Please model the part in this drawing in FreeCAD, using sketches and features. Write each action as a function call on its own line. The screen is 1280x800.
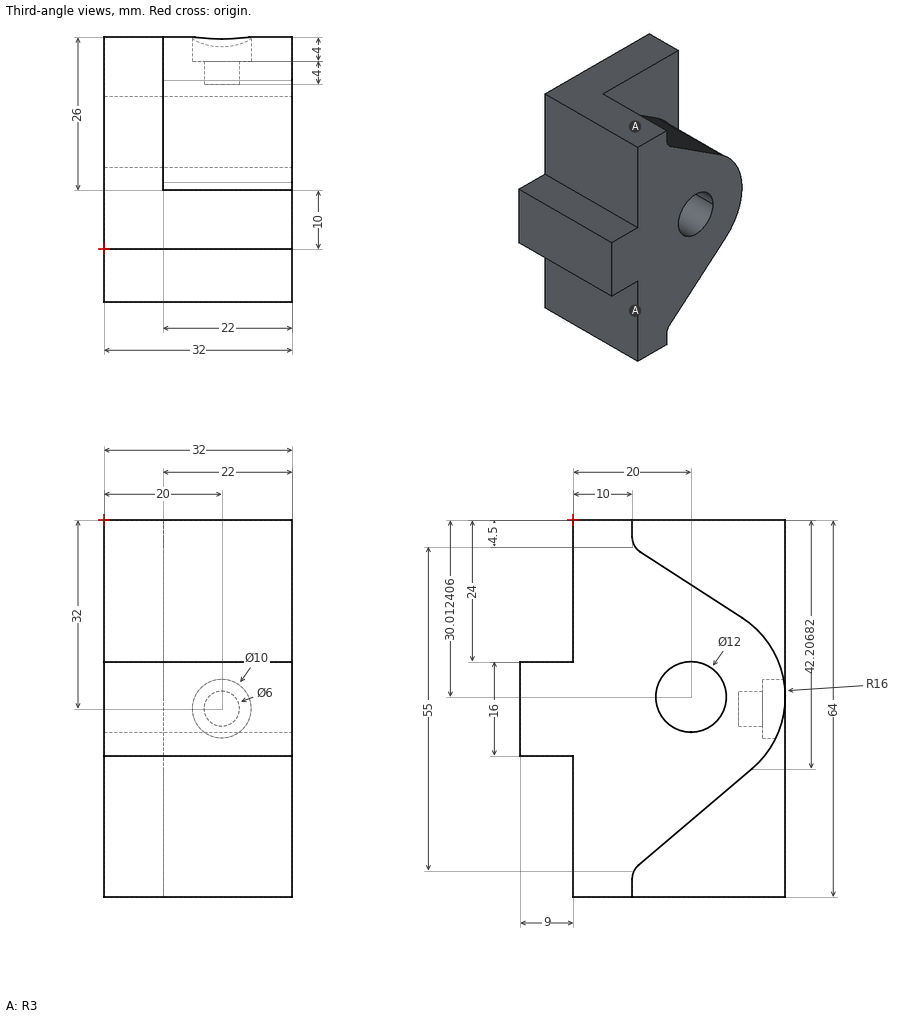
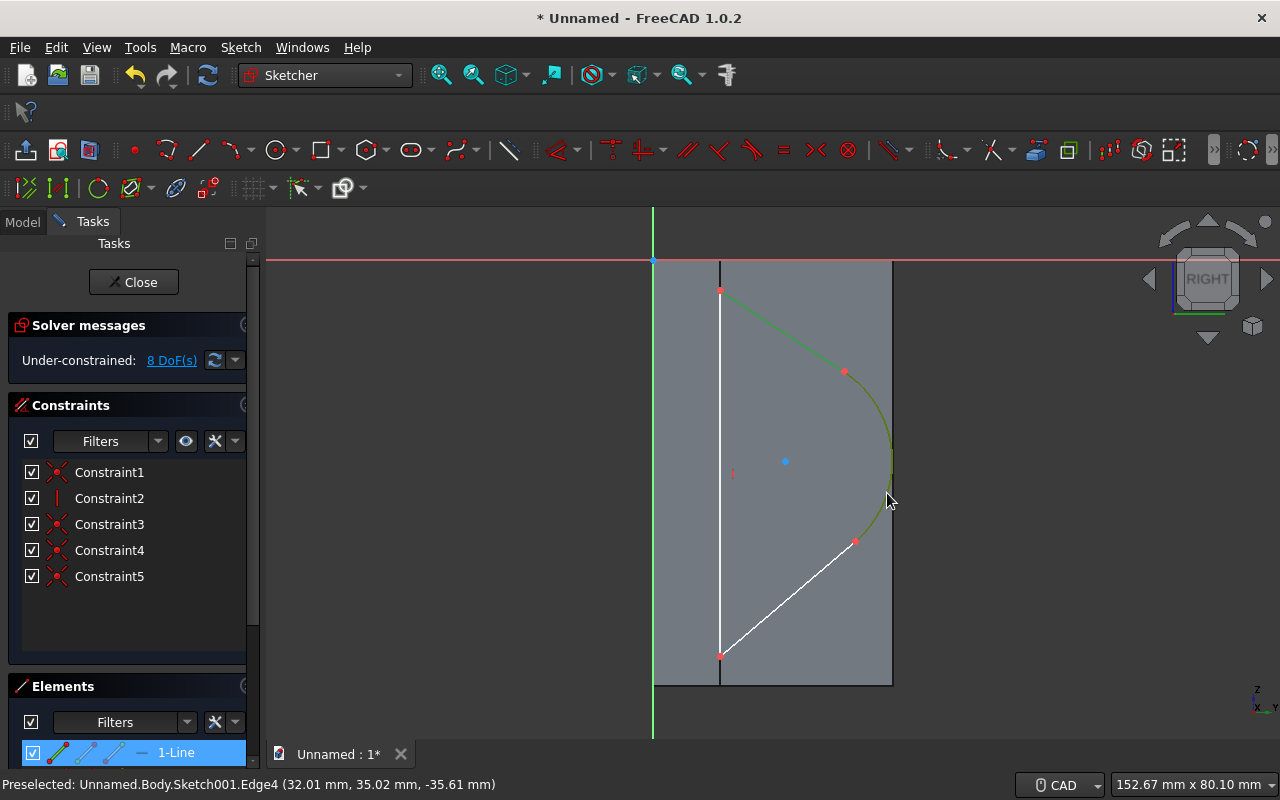
key(t)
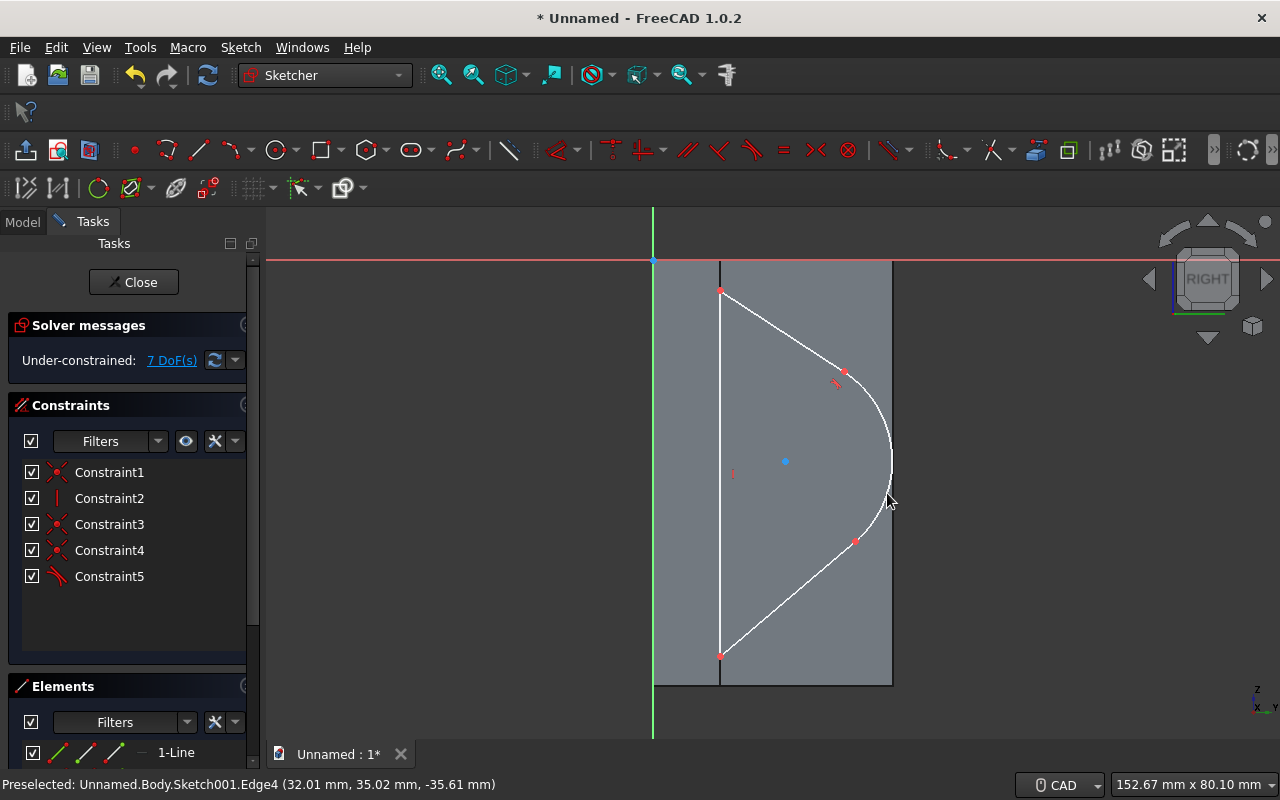
click(760, 623)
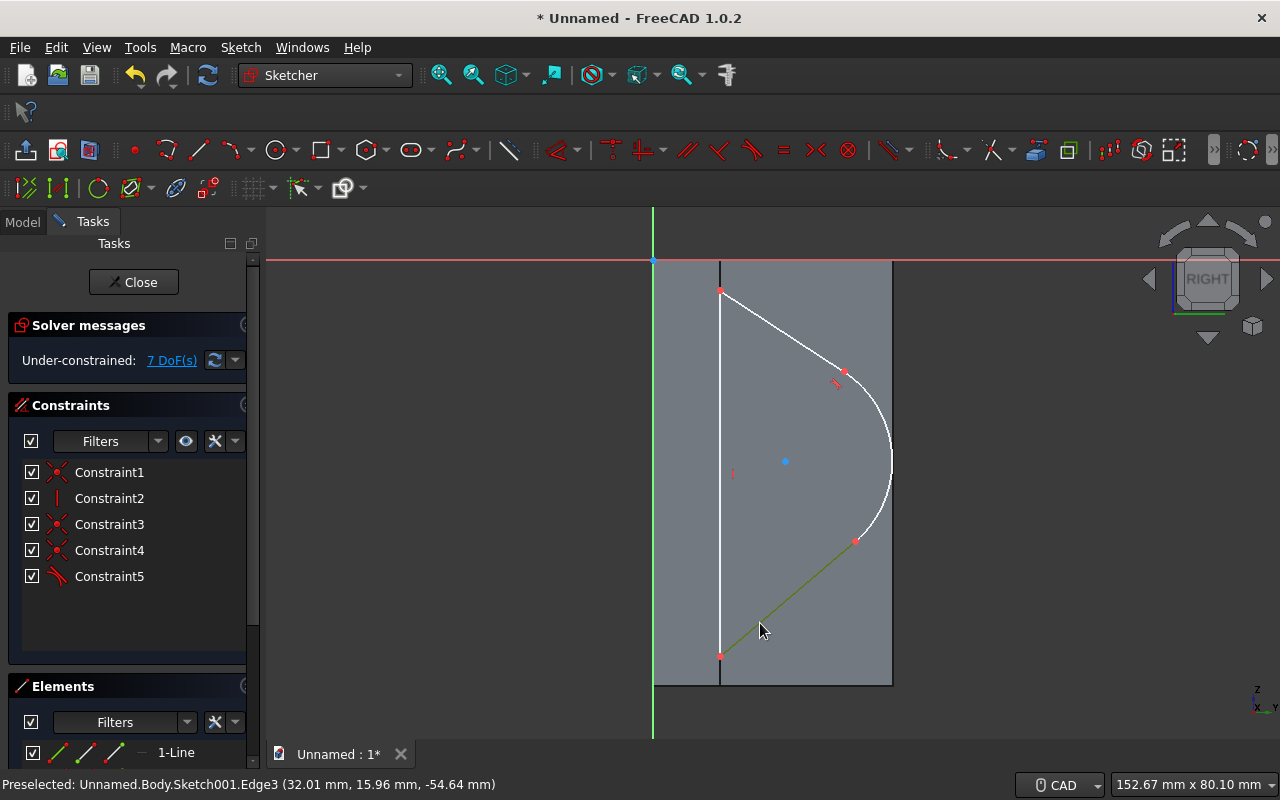
click(887, 493)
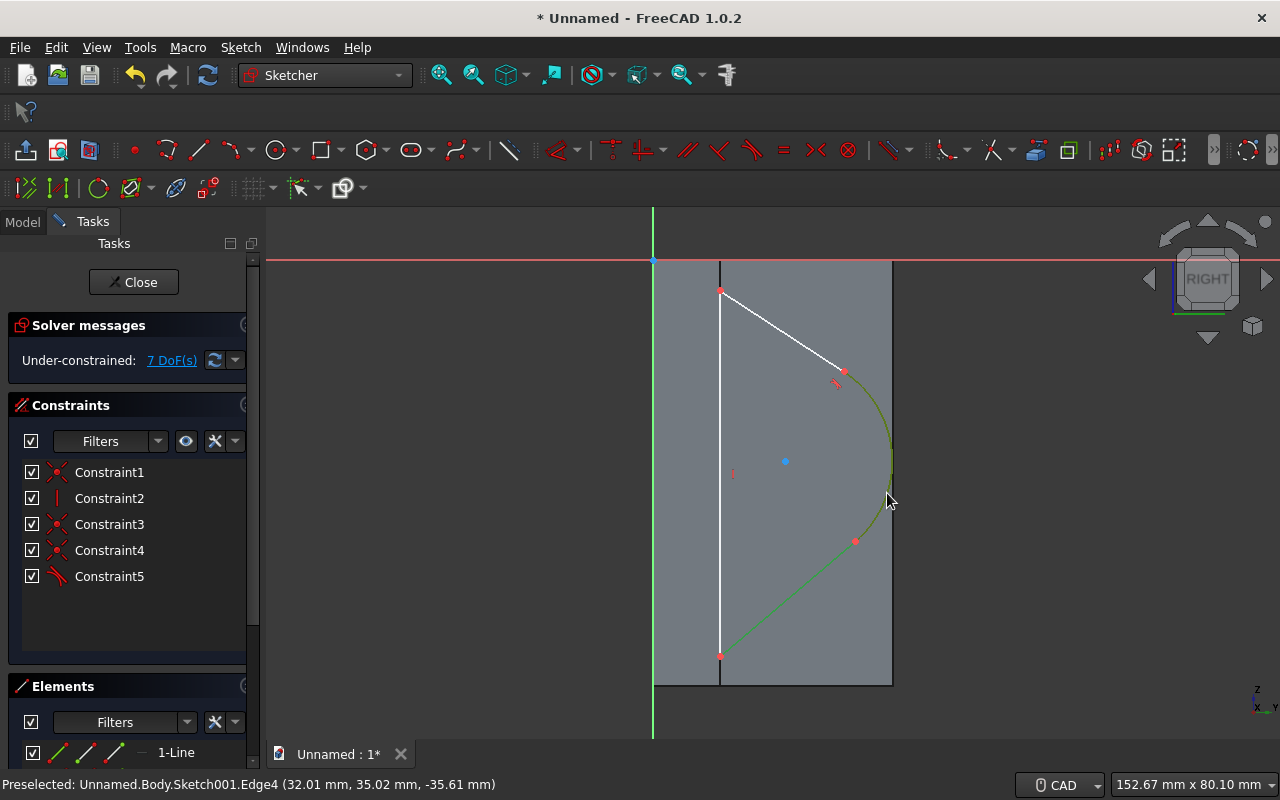
key(t)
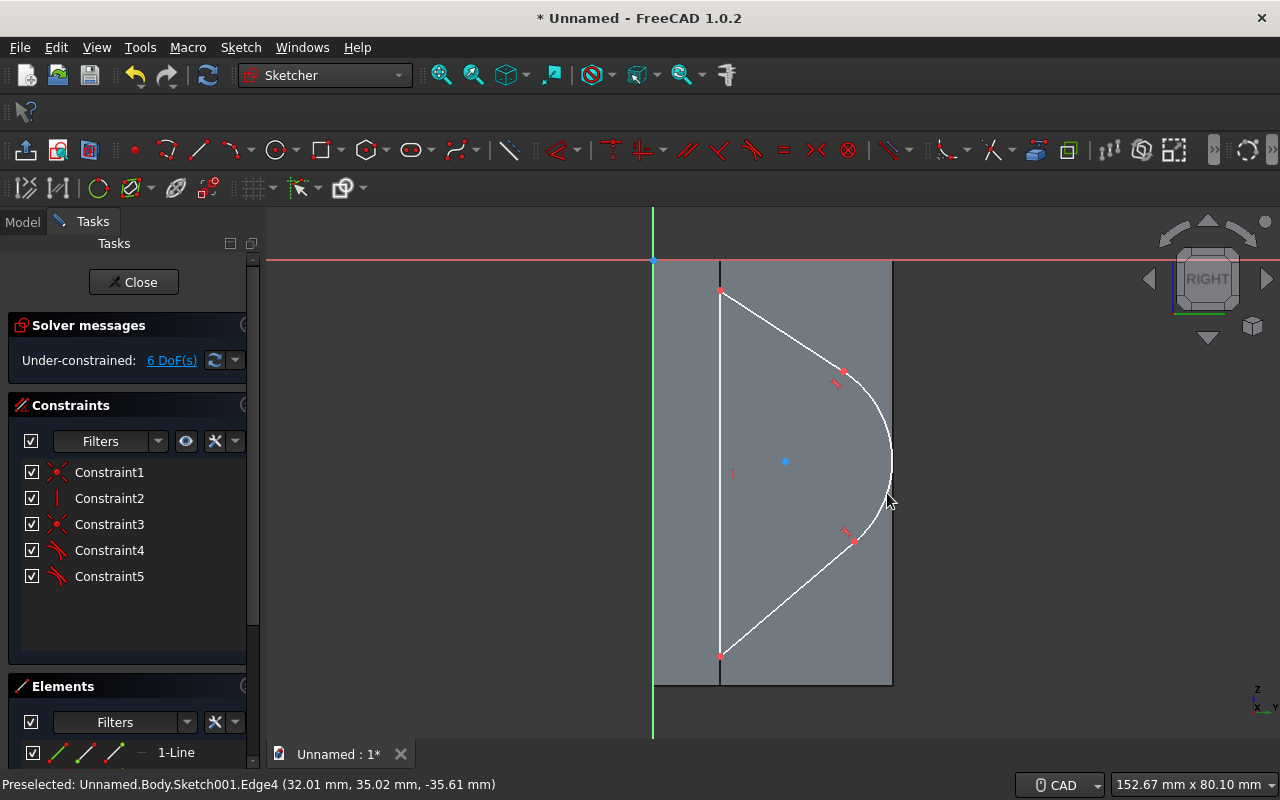
key(d)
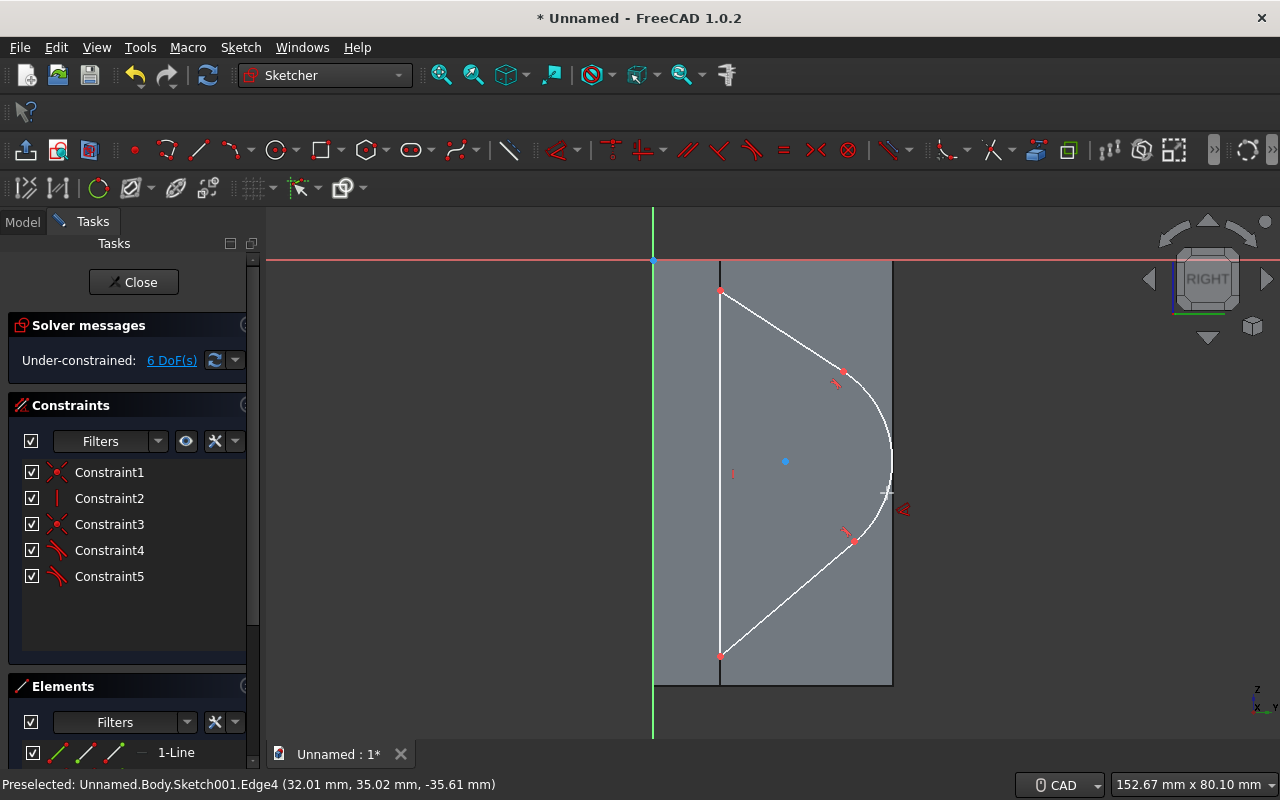
click(887, 493)
click(918, 503)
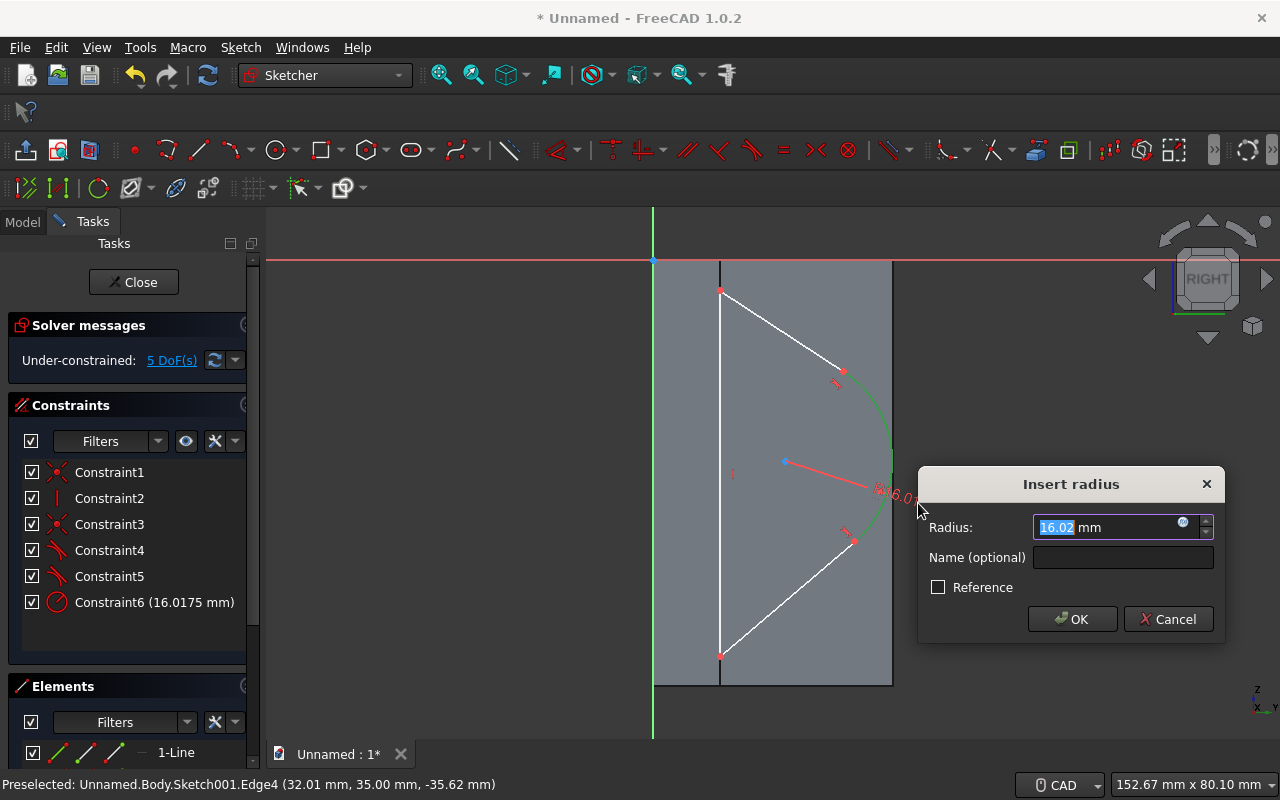
text(16)
key(Return)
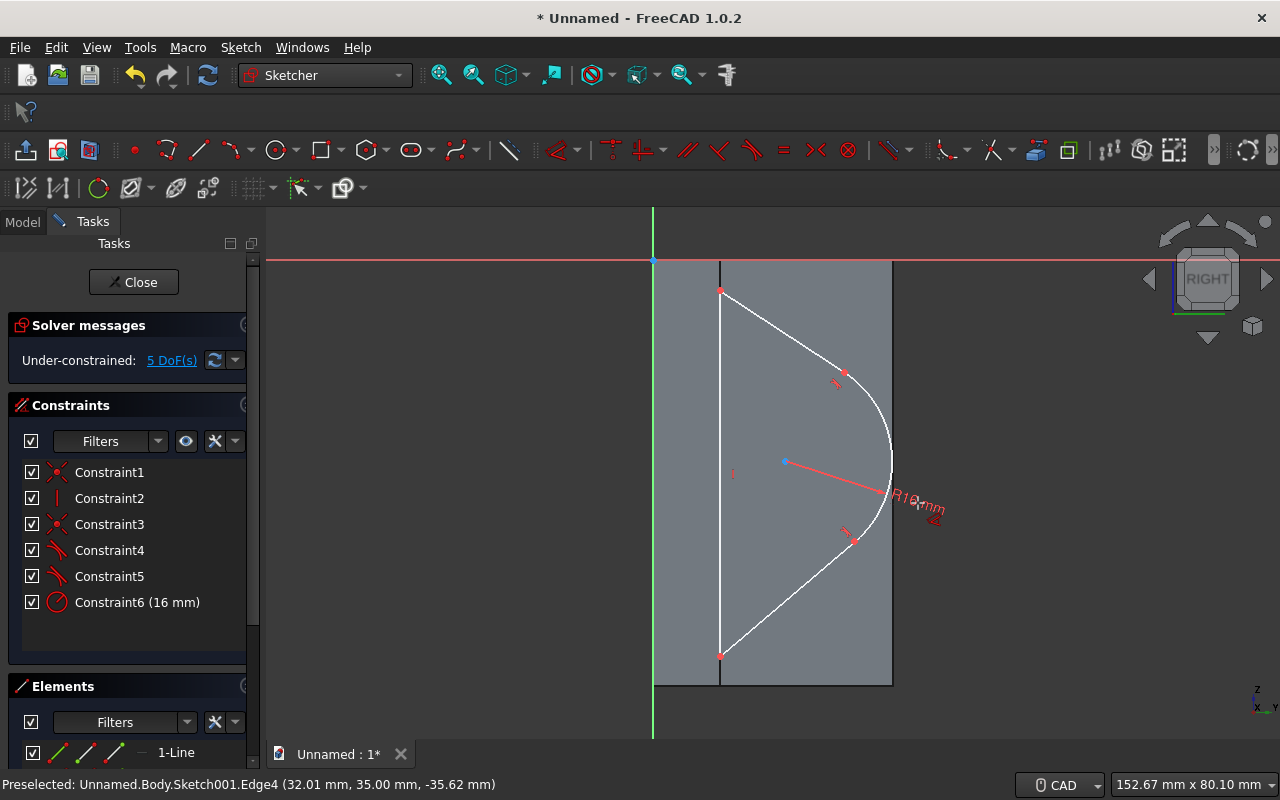
click(720, 401)
click(686, 474)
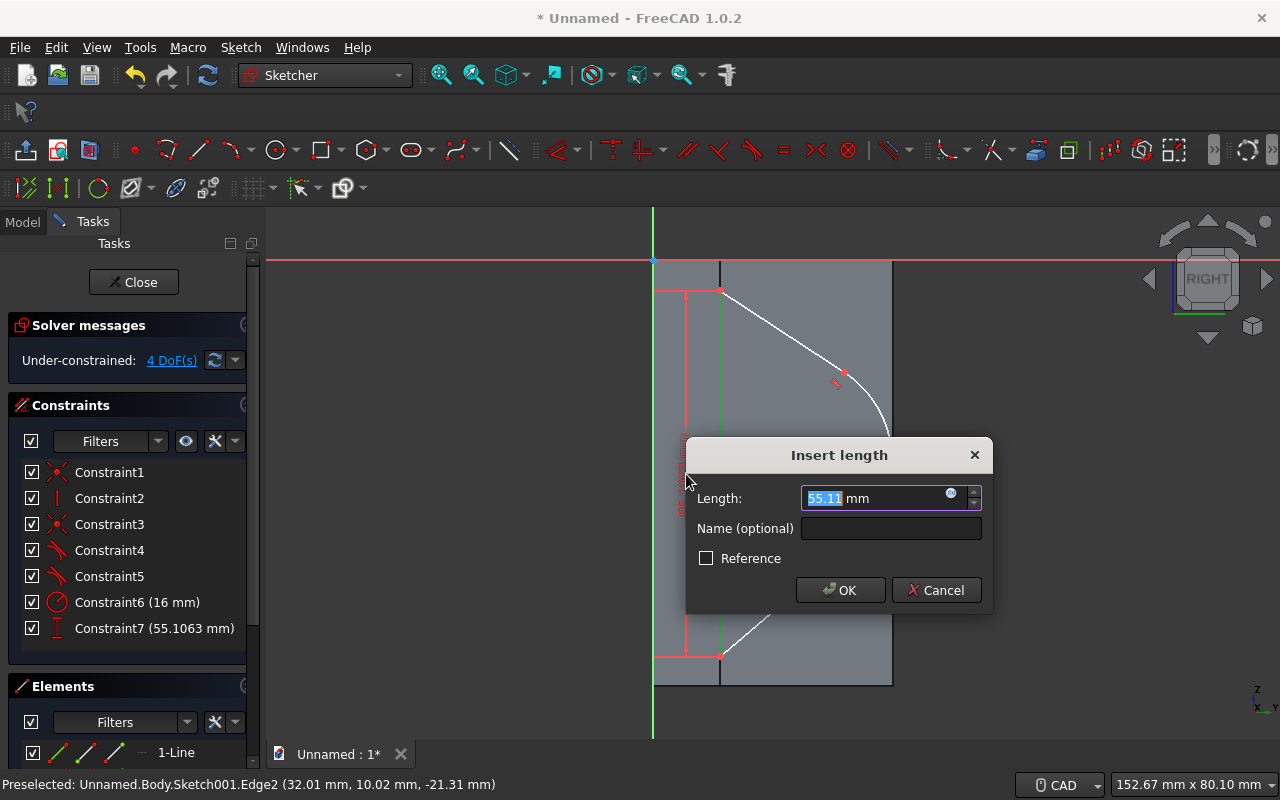
text(55)
key(Return)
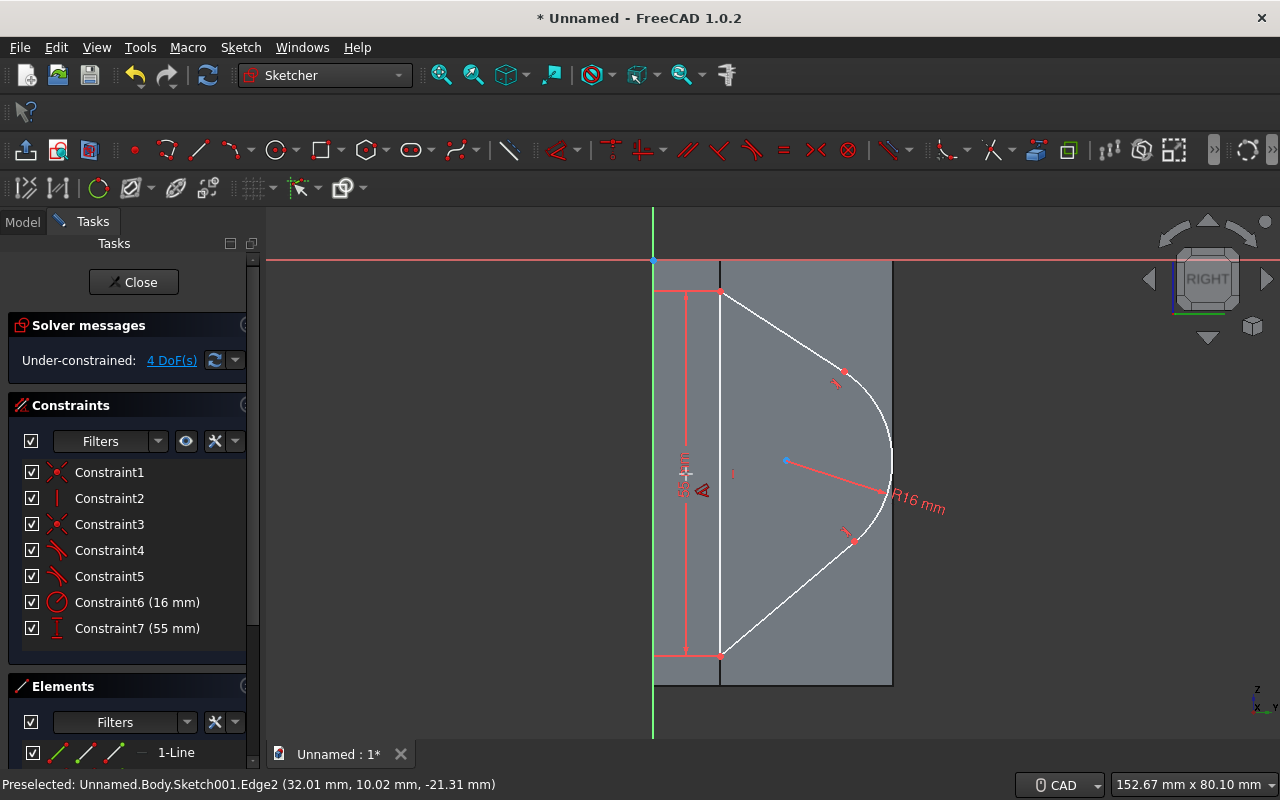
click(720, 291)
click(687, 325)